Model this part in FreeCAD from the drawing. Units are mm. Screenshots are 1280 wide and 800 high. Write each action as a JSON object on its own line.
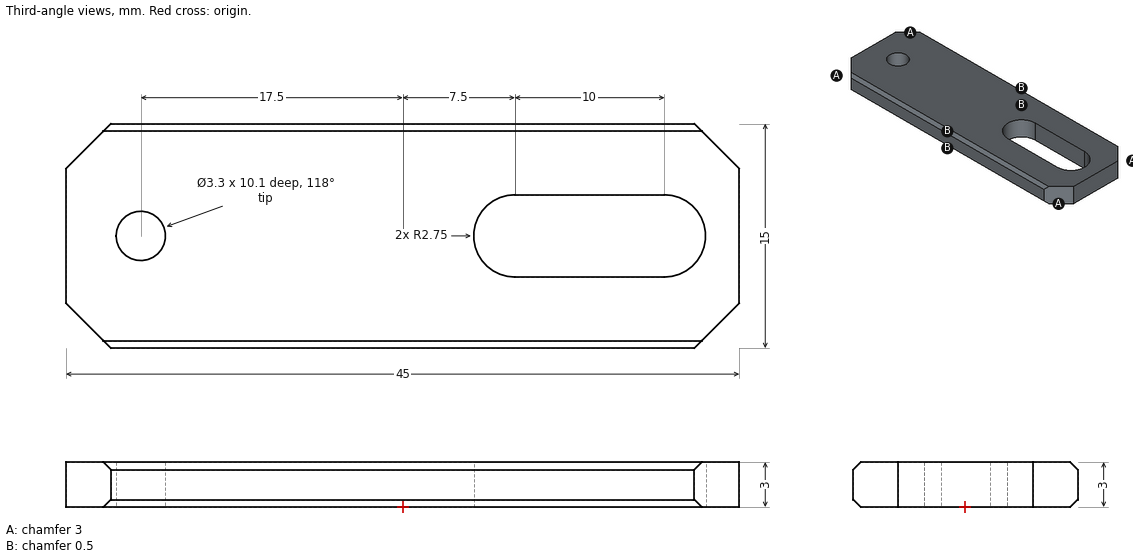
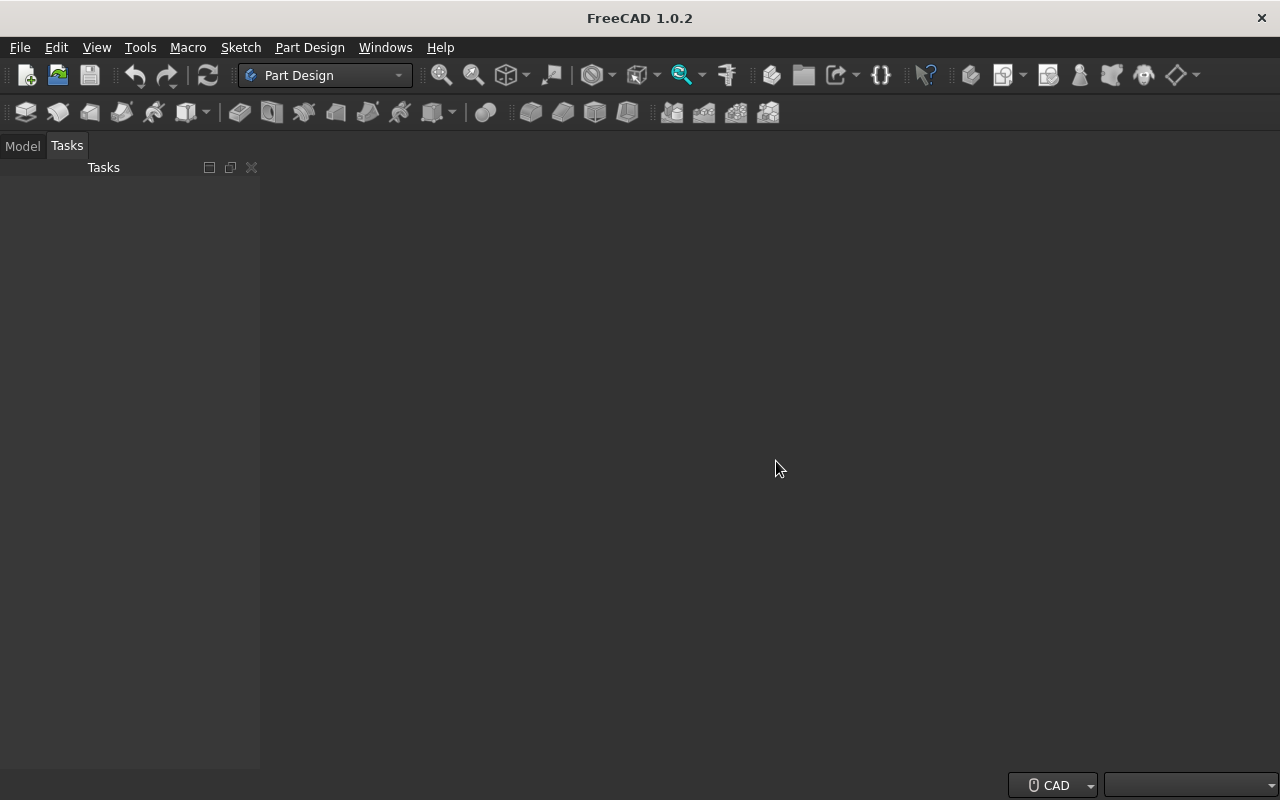
{"action": "left_click", "coordinate": [26, 76]}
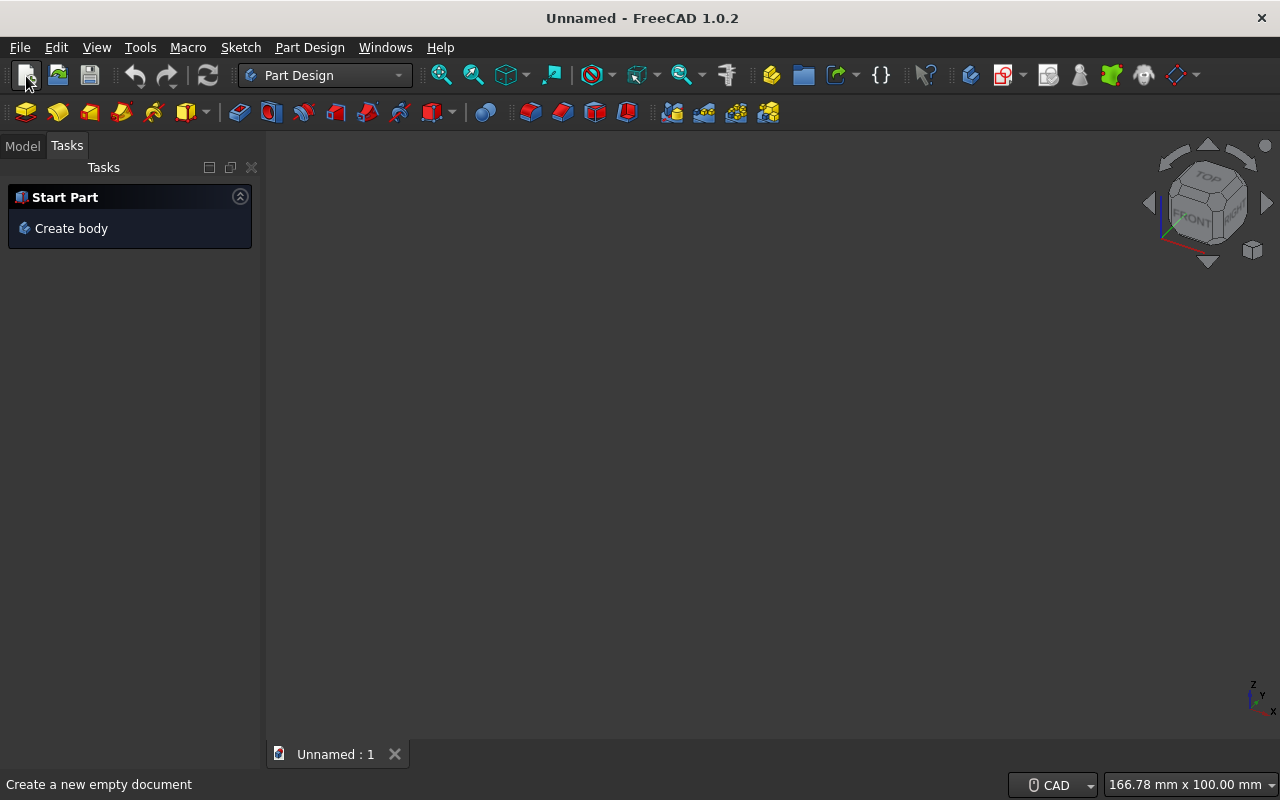
{"action": "left_click", "coordinate": [1004, 76]}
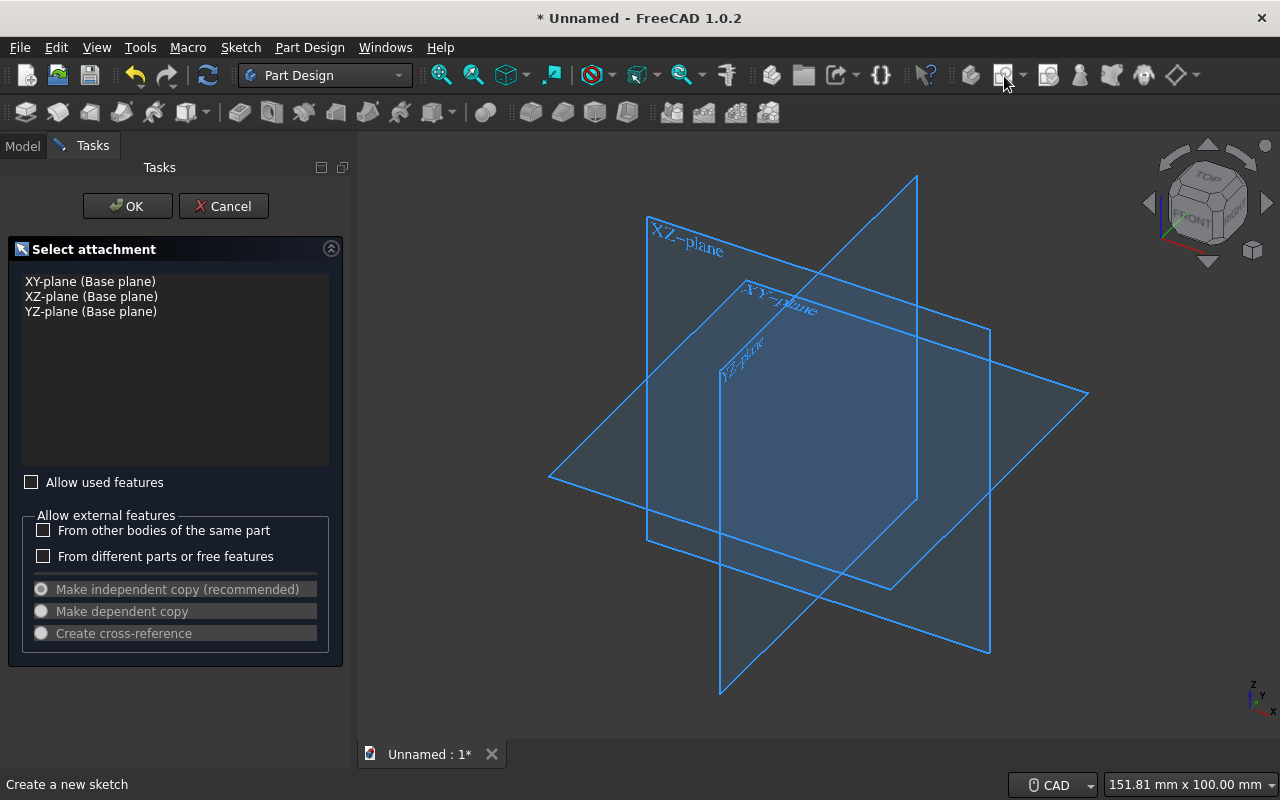
{"action": "left_click", "coordinate": [82, 282]}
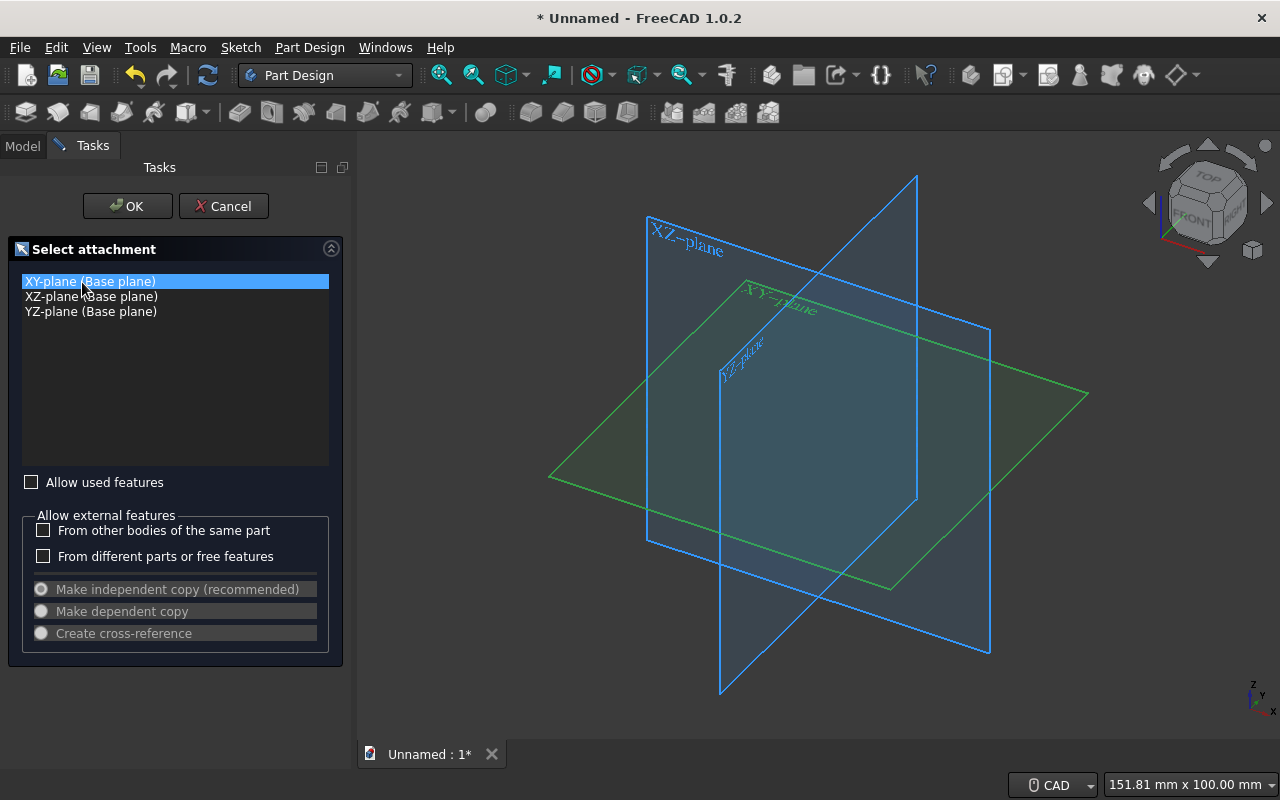
{"action": "left_click", "coordinate": [128, 206]}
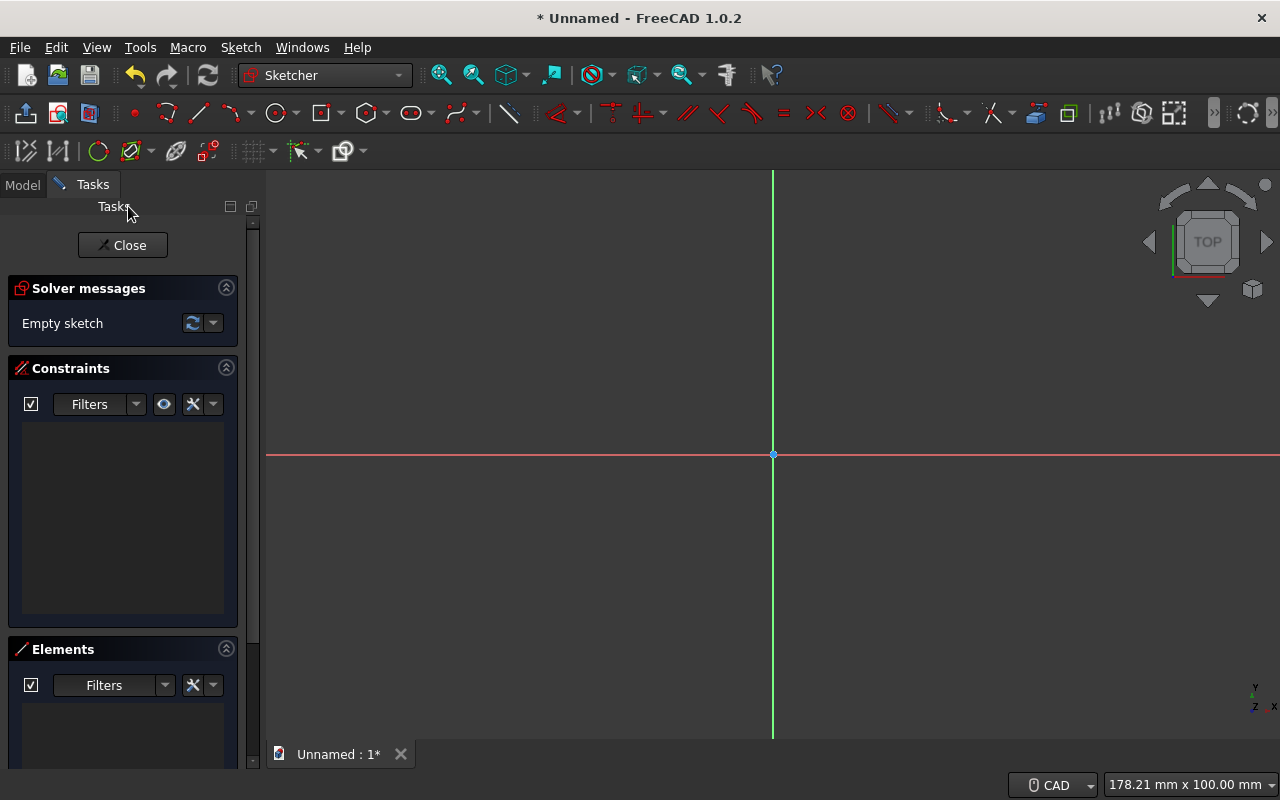
{"action": "scroll", "coordinate": [829, 455], "scroll_direction": "up", "scroll_amount": 4}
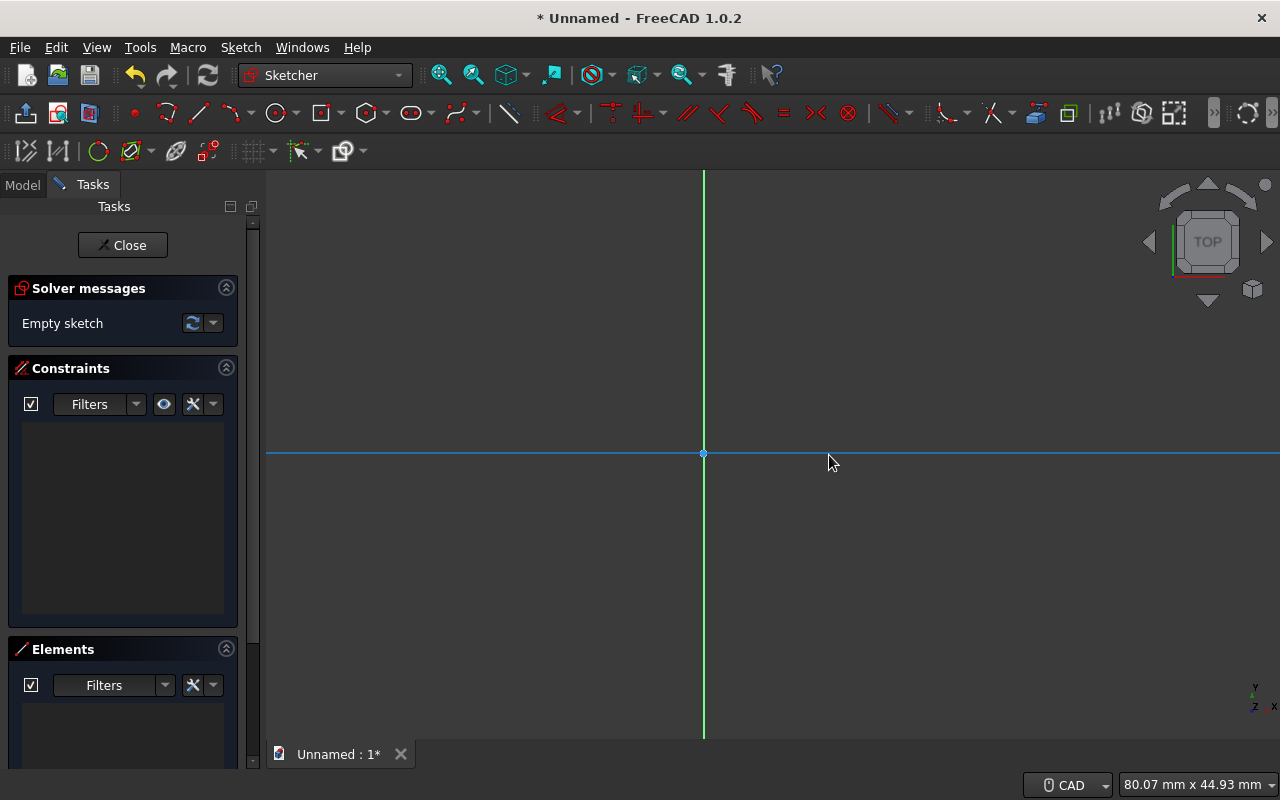
{"action": "left_click", "coordinate": [322, 114]}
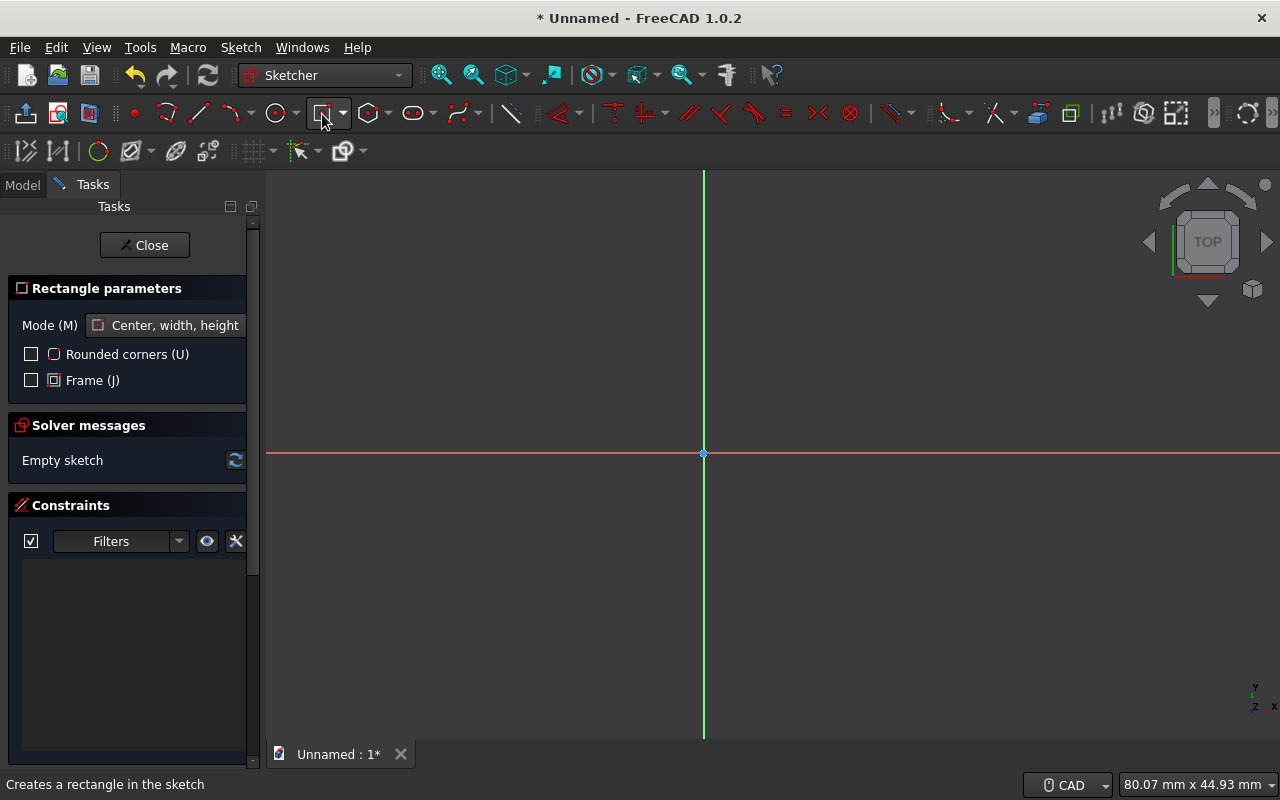
{"action": "left_click", "coordinate": [704, 453]}
{"action": "mouse_move", "coordinate": [989, 358]}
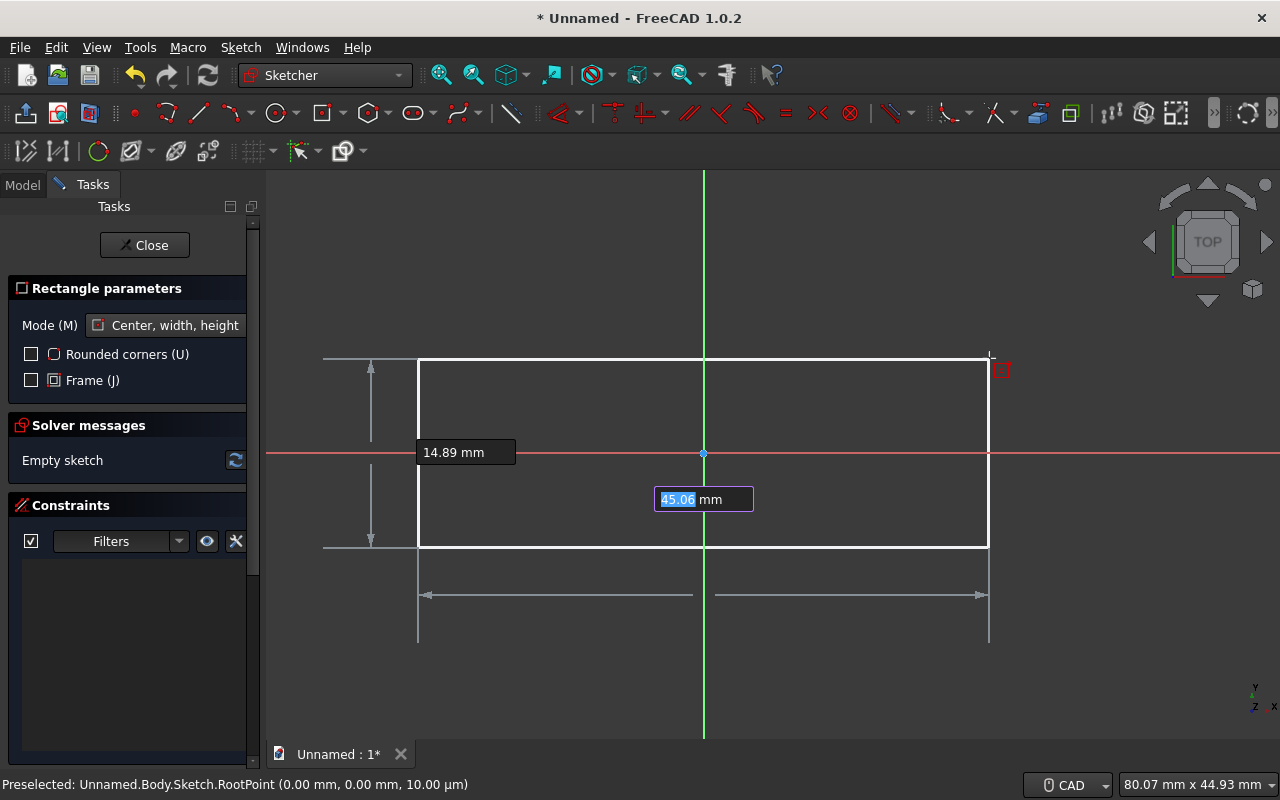
{"action": "type", "text": "45"}
{"action": "key", "text": "Tab"}
{"action": "type", "text": "15"}
{"action": "key", "text": "Return"}
{"action": "key", "text": "Escape"}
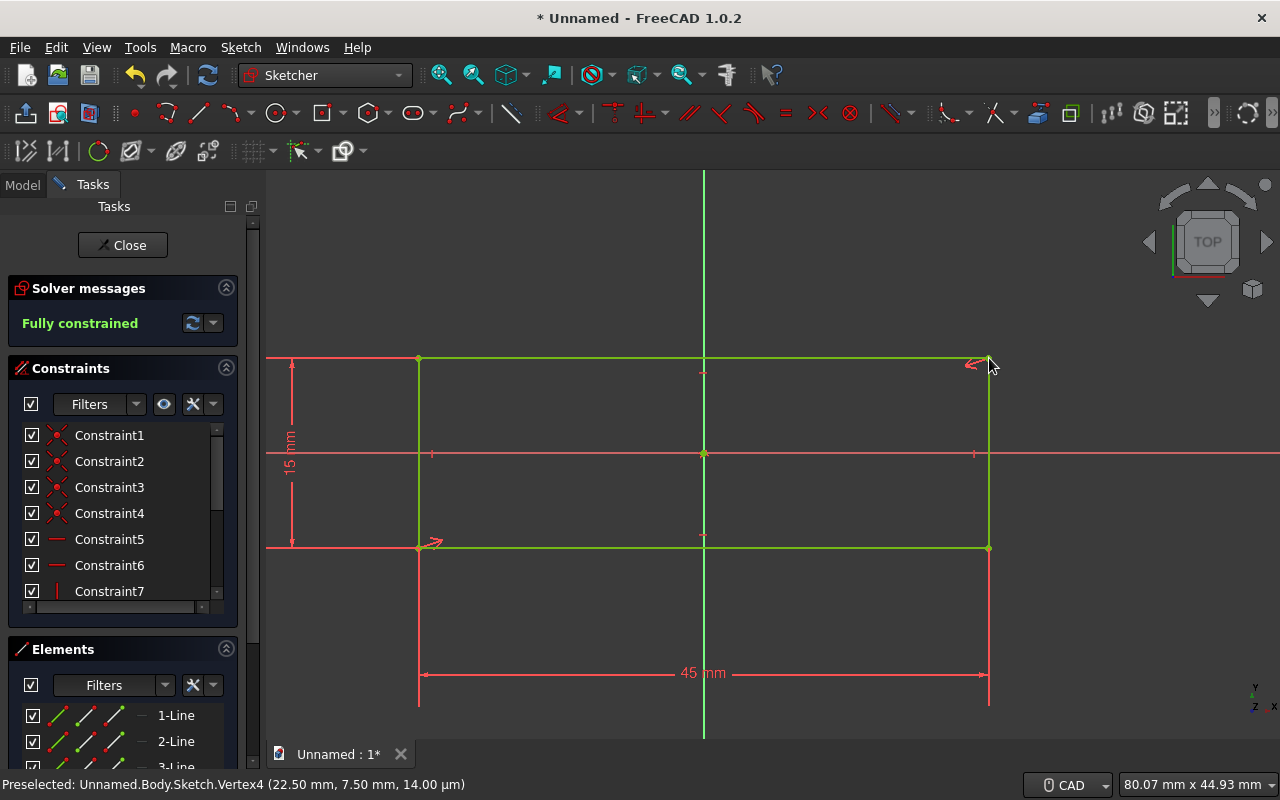
{"action": "left_click", "coordinate": [123, 245]}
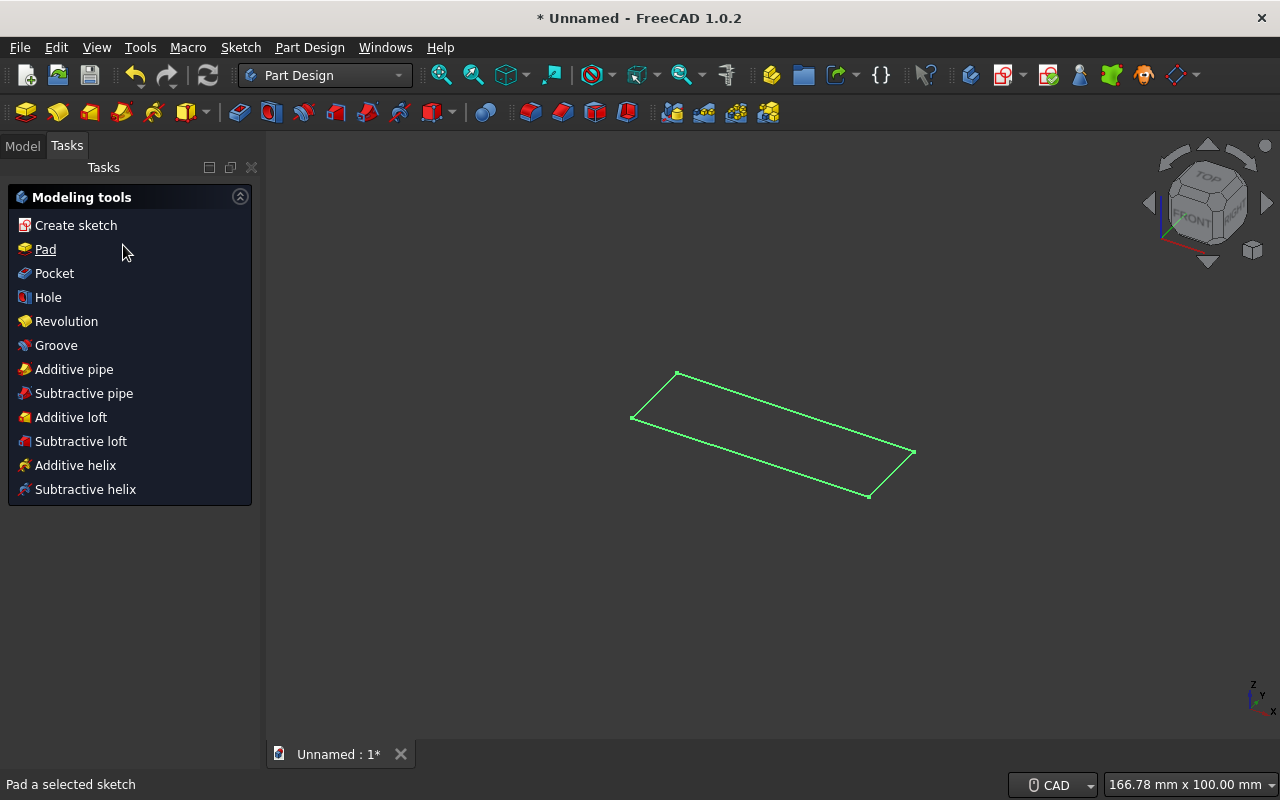
{"action": "left_click", "coordinate": [26, 112]}